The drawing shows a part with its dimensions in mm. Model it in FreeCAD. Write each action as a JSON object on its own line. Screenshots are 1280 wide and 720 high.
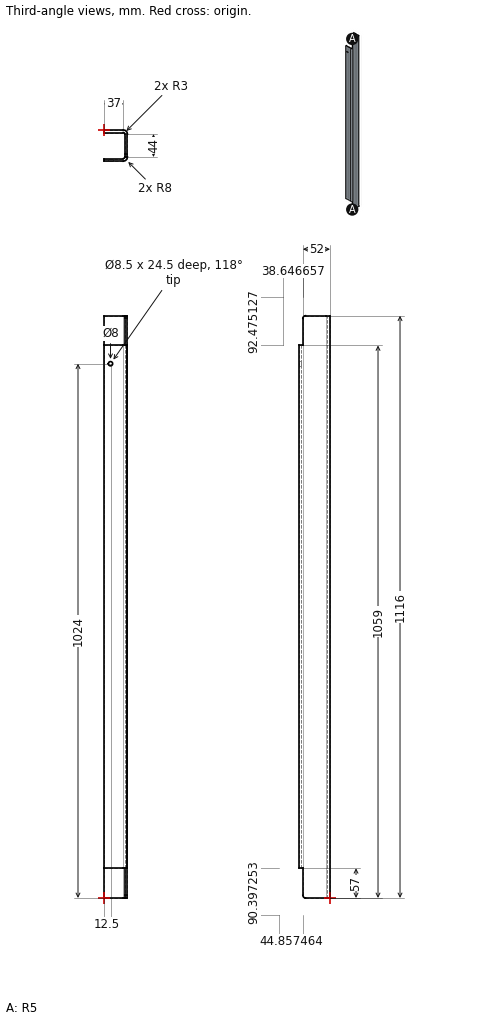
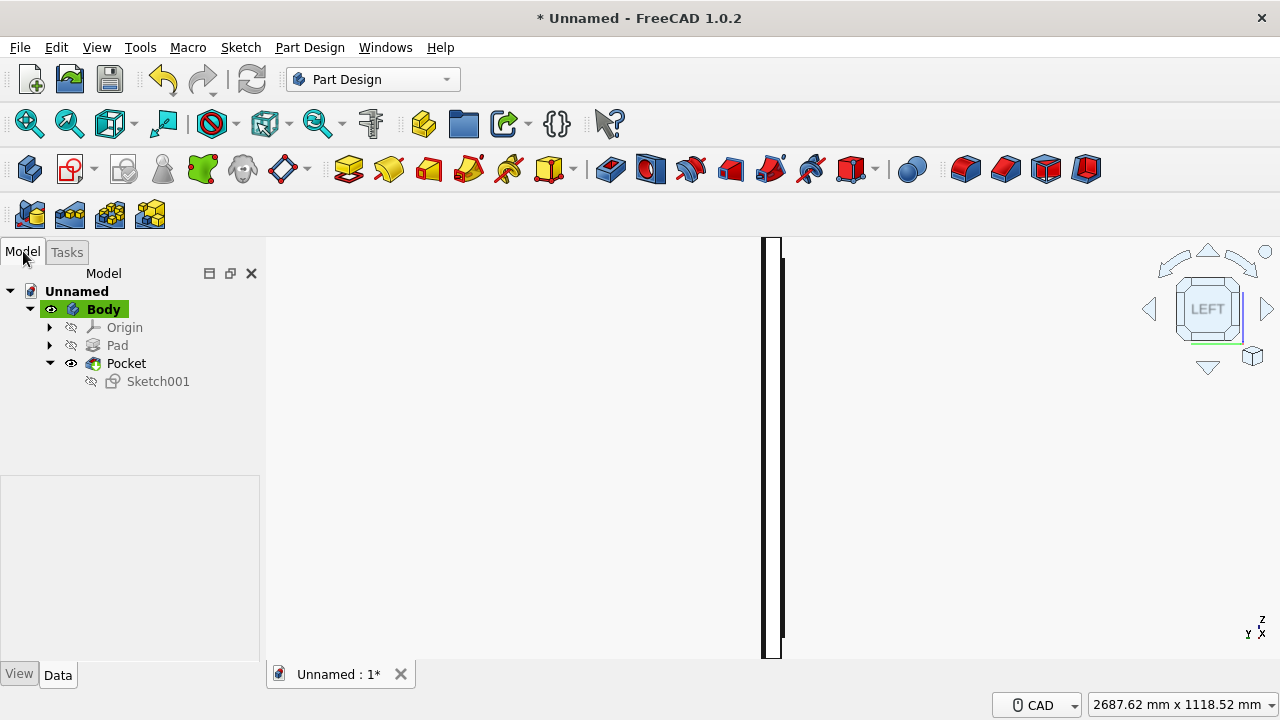
{"action": "left_click", "coordinate": [50, 327]}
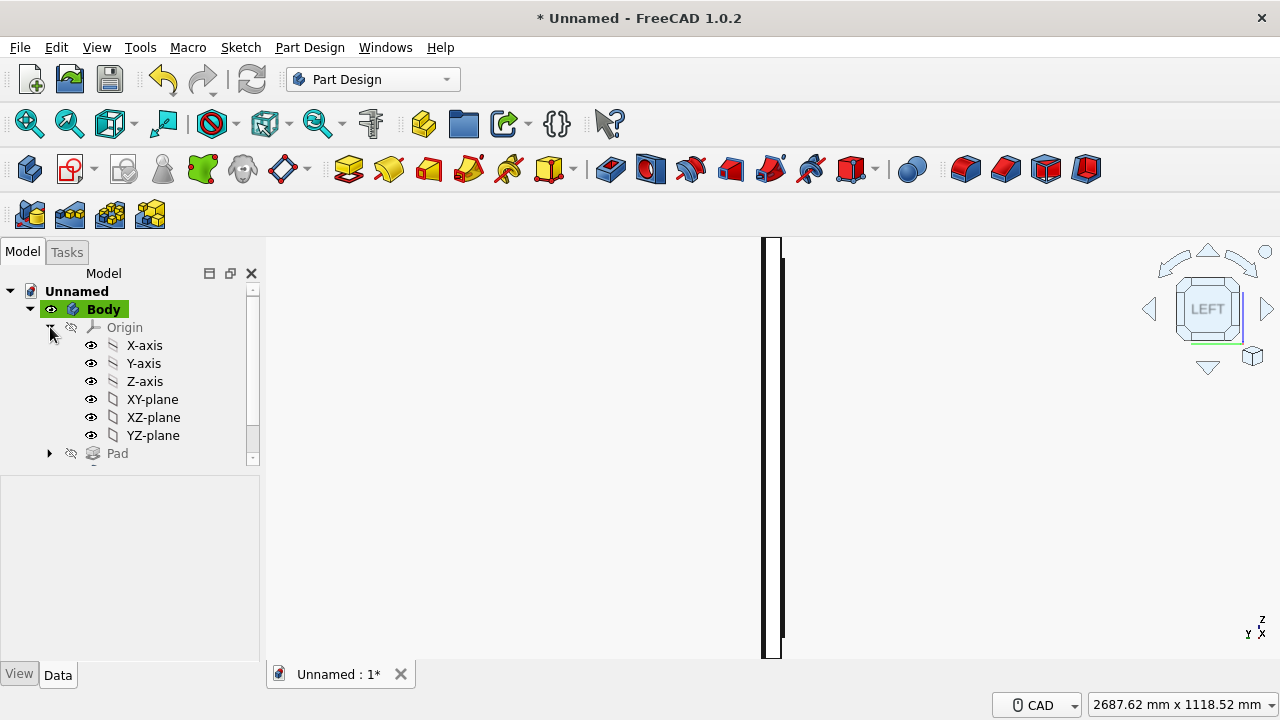
{"action": "left_click", "coordinate": [136, 417]}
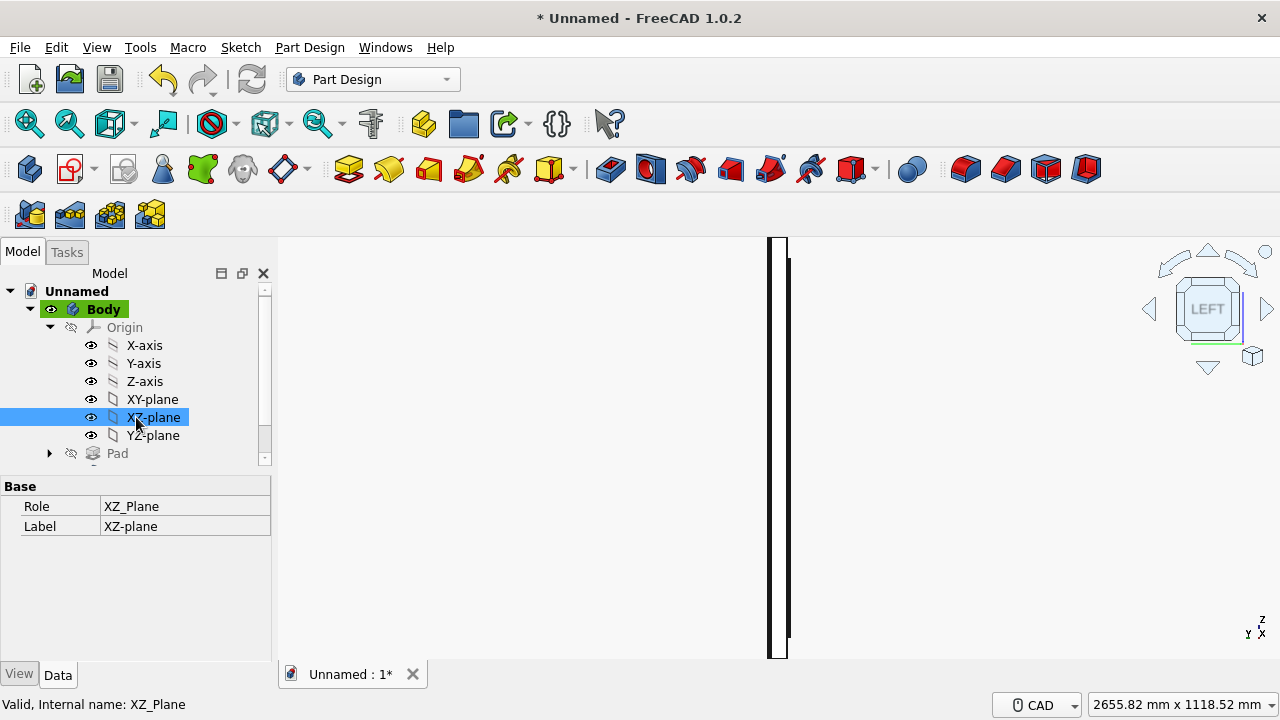
{"action": "left_click", "coordinate": [284, 170]}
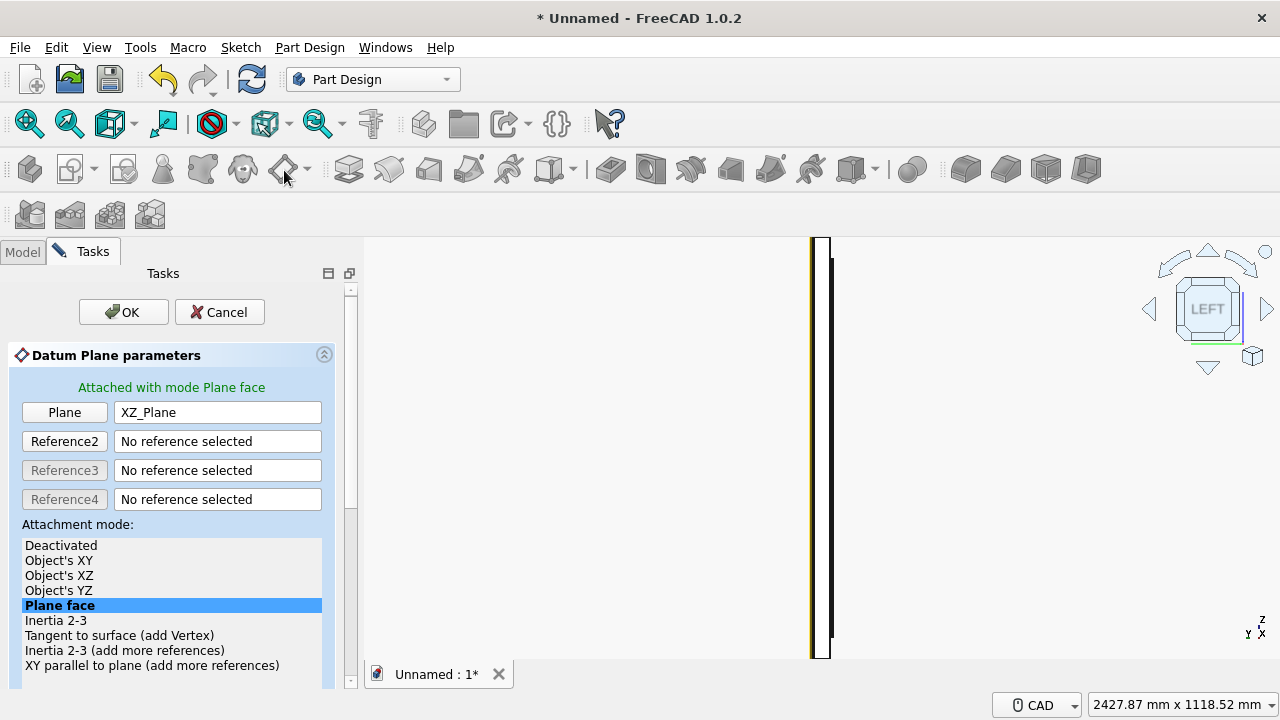
{"action": "scroll", "coordinate": [351, 486], "scroll_direction": "down", "scroll_amount": 4}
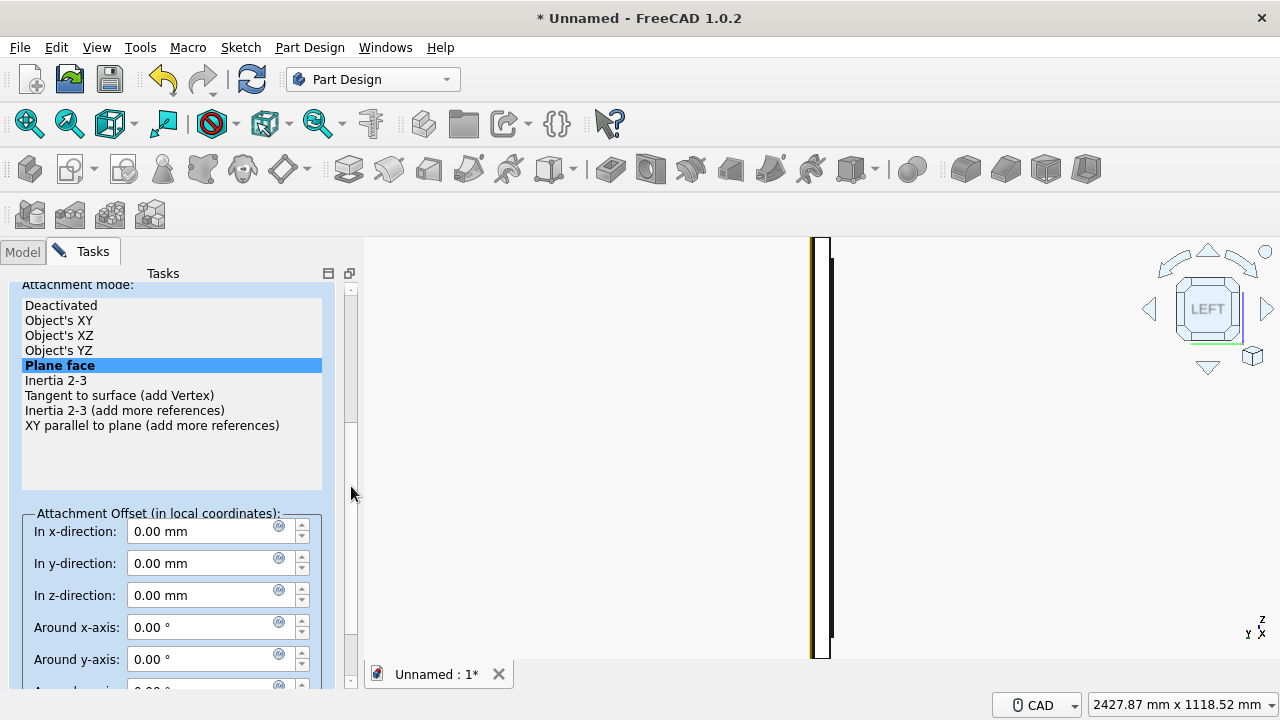
{"action": "triple_click", "coordinate": [210, 595]}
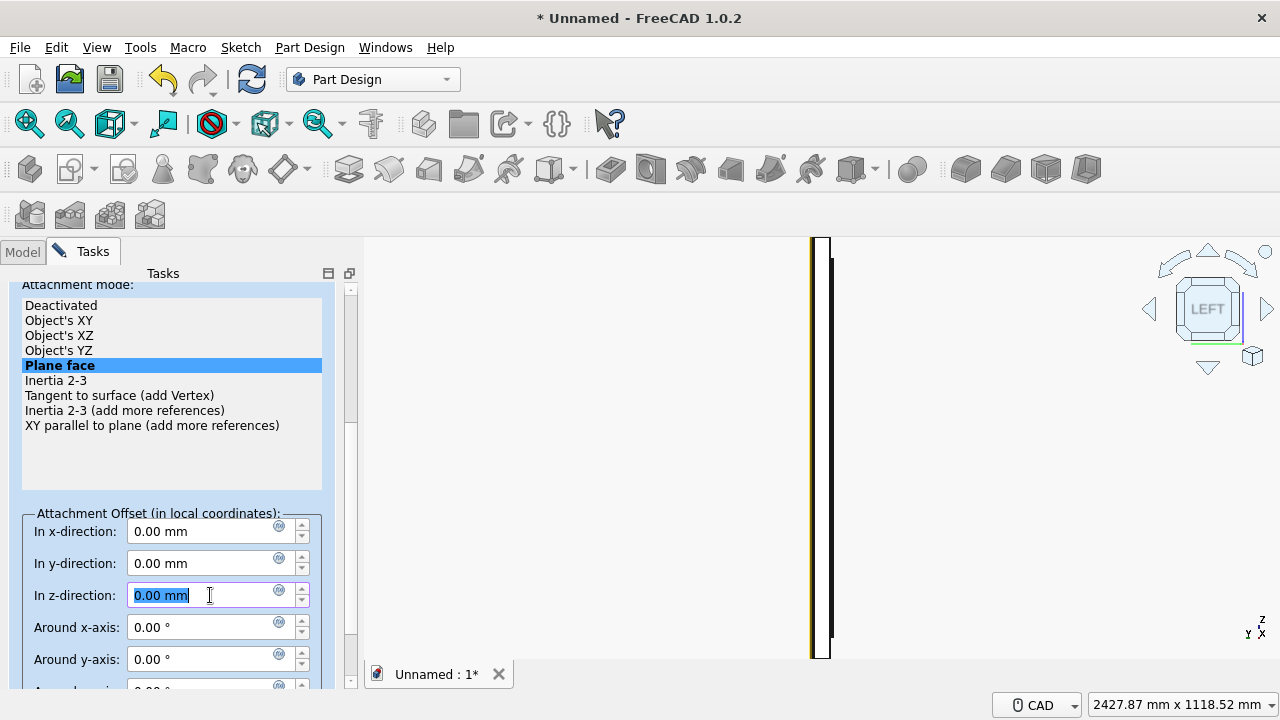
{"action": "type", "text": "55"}
{"action": "key", "text": "Tab"}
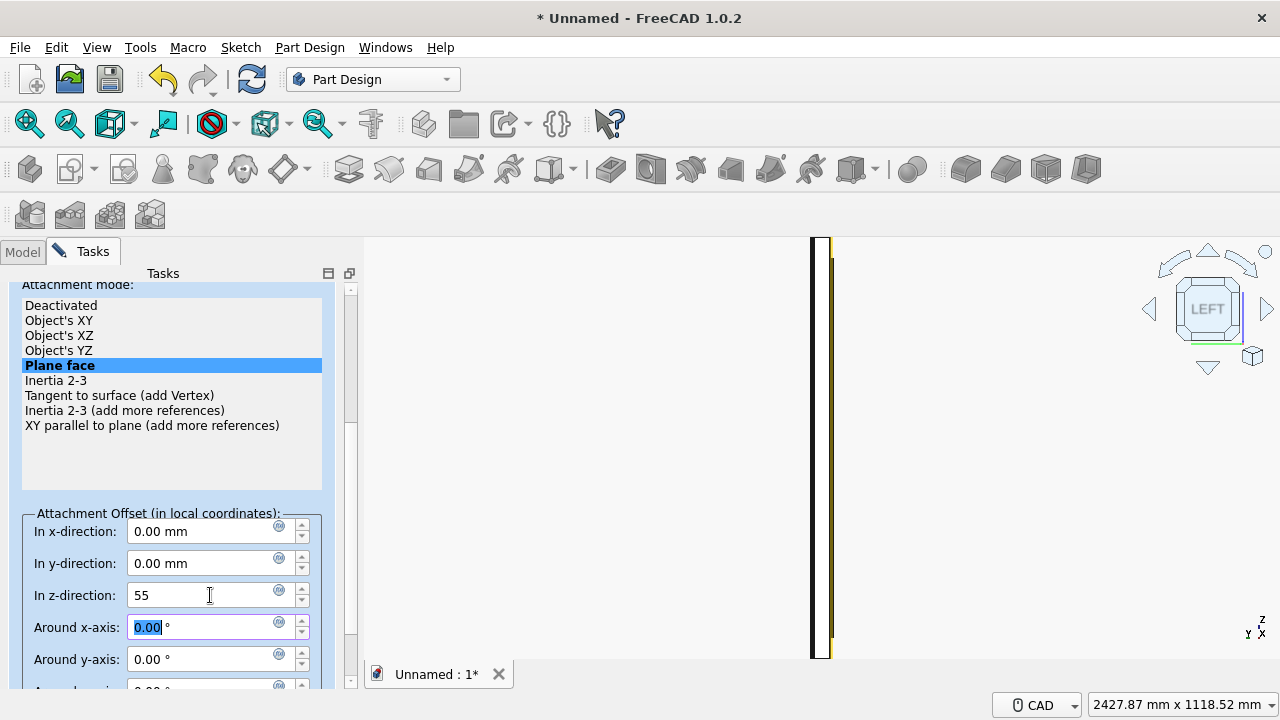
{"action": "scroll", "coordinate": [351, 486], "scroll_direction": "up", "scroll_amount": 5}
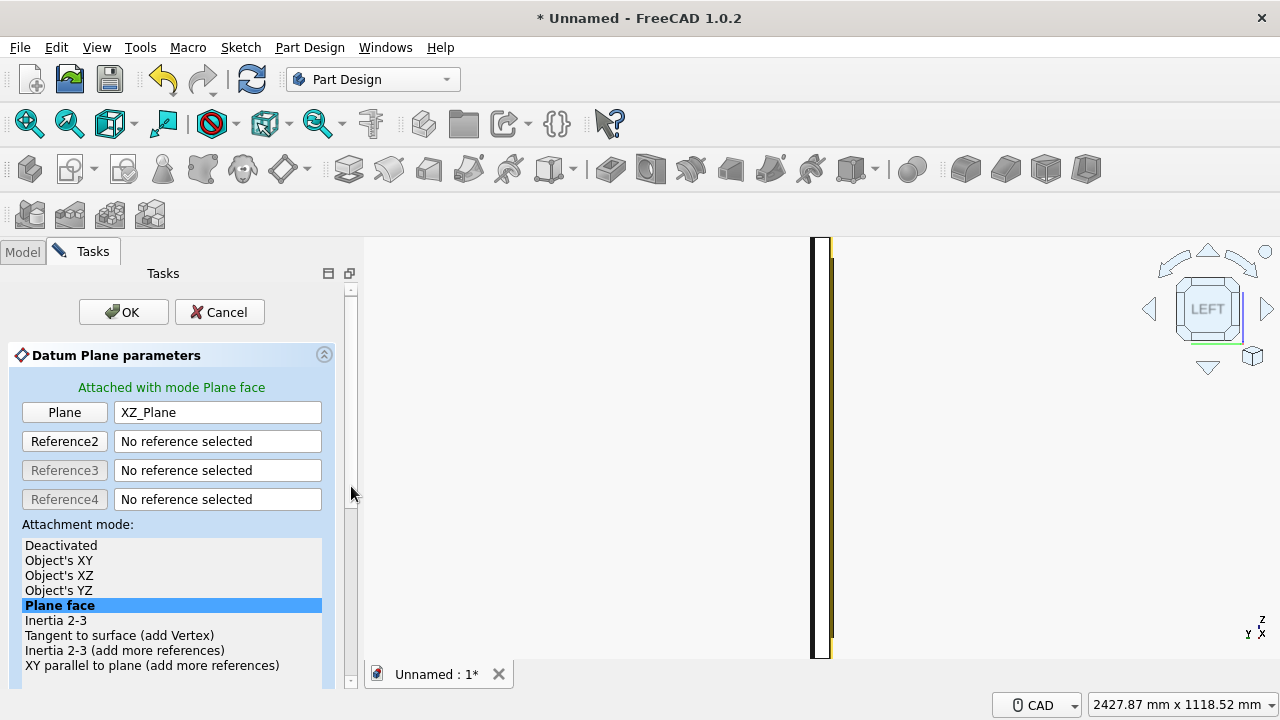
{"action": "left_click", "coordinate": [124, 312]}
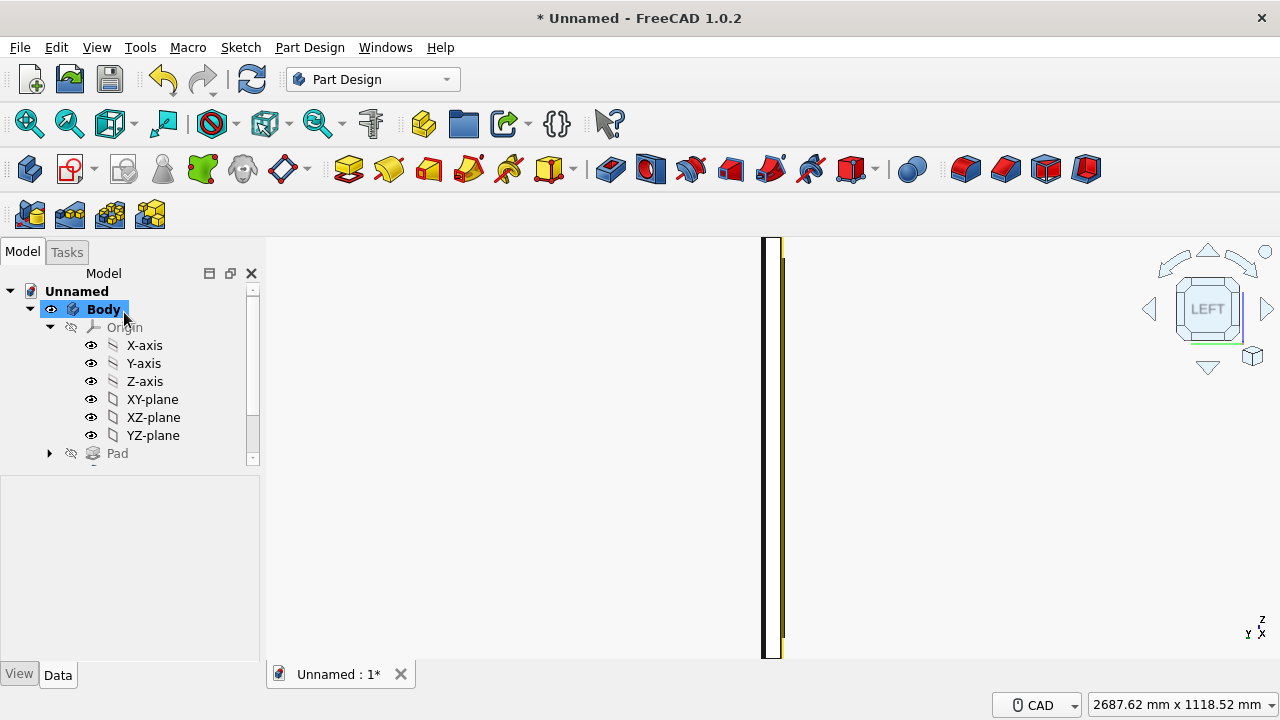
{"action": "scroll", "coordinate": [100, 377], "scroll_direction": "down", "scroll_amount": 3}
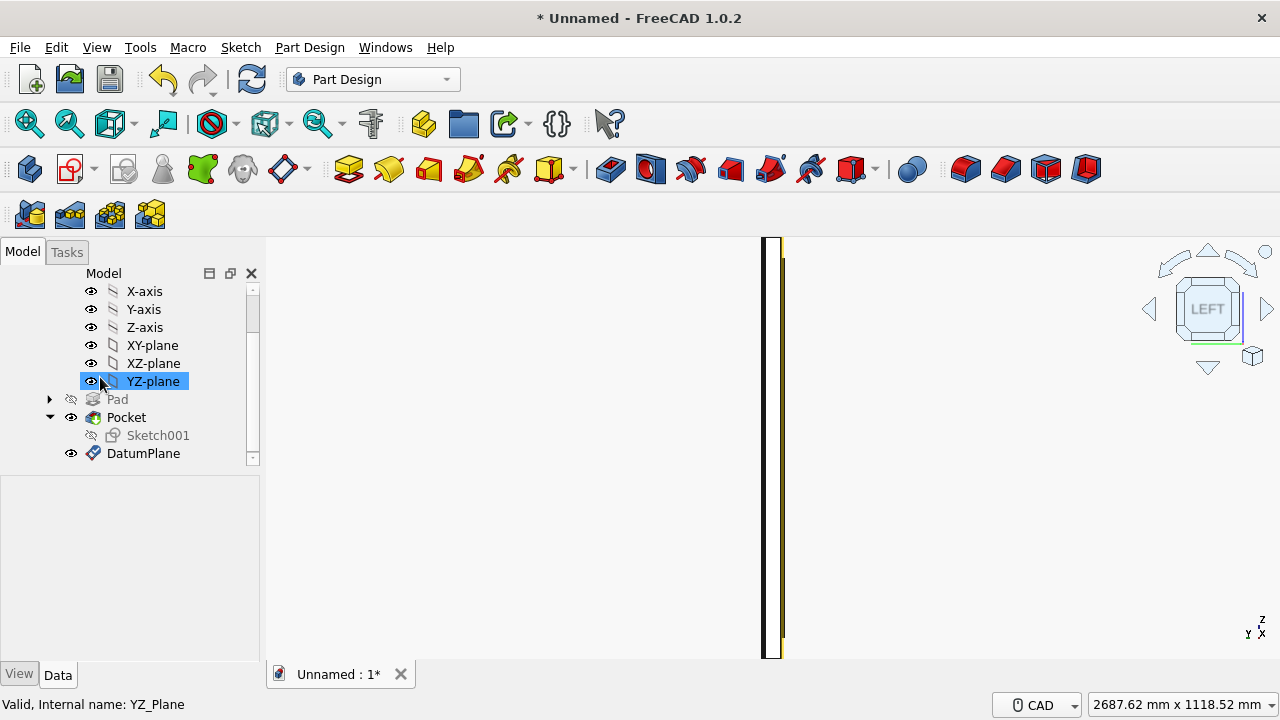
{"action": "left_click", "coordinate": [116, 453]}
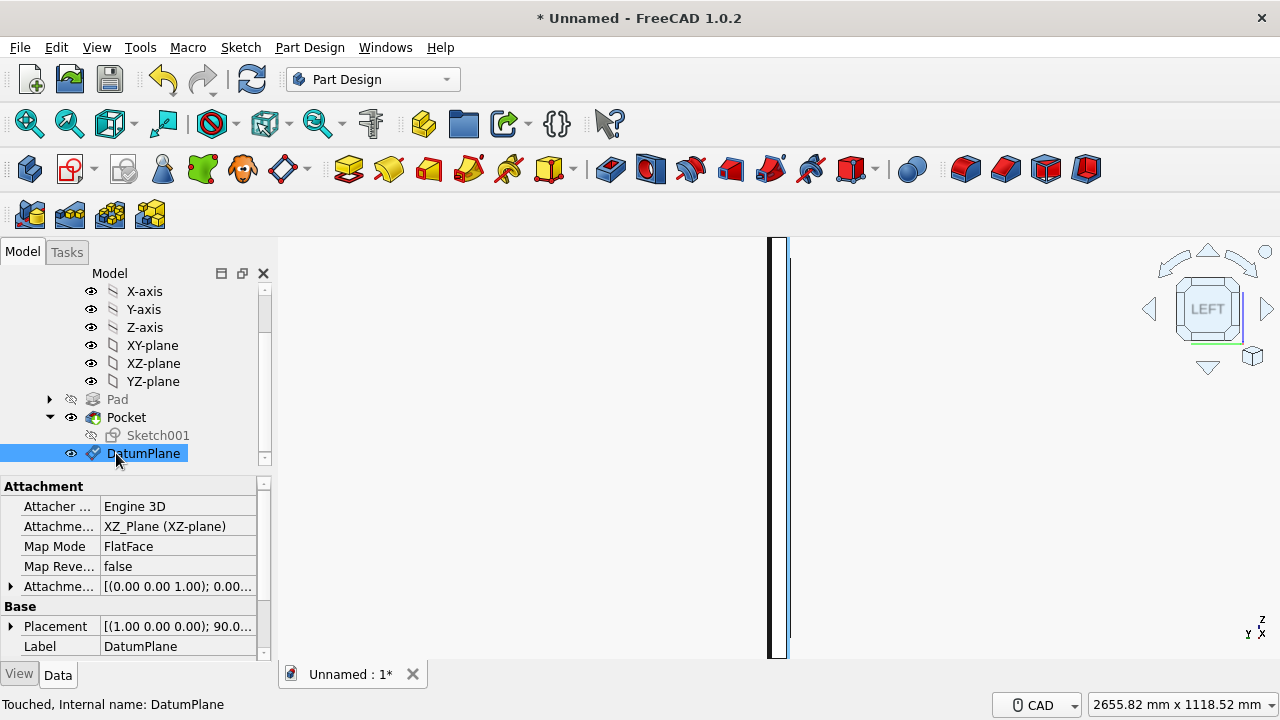
{"action": "left_click", "coordinate": [70, 170]}